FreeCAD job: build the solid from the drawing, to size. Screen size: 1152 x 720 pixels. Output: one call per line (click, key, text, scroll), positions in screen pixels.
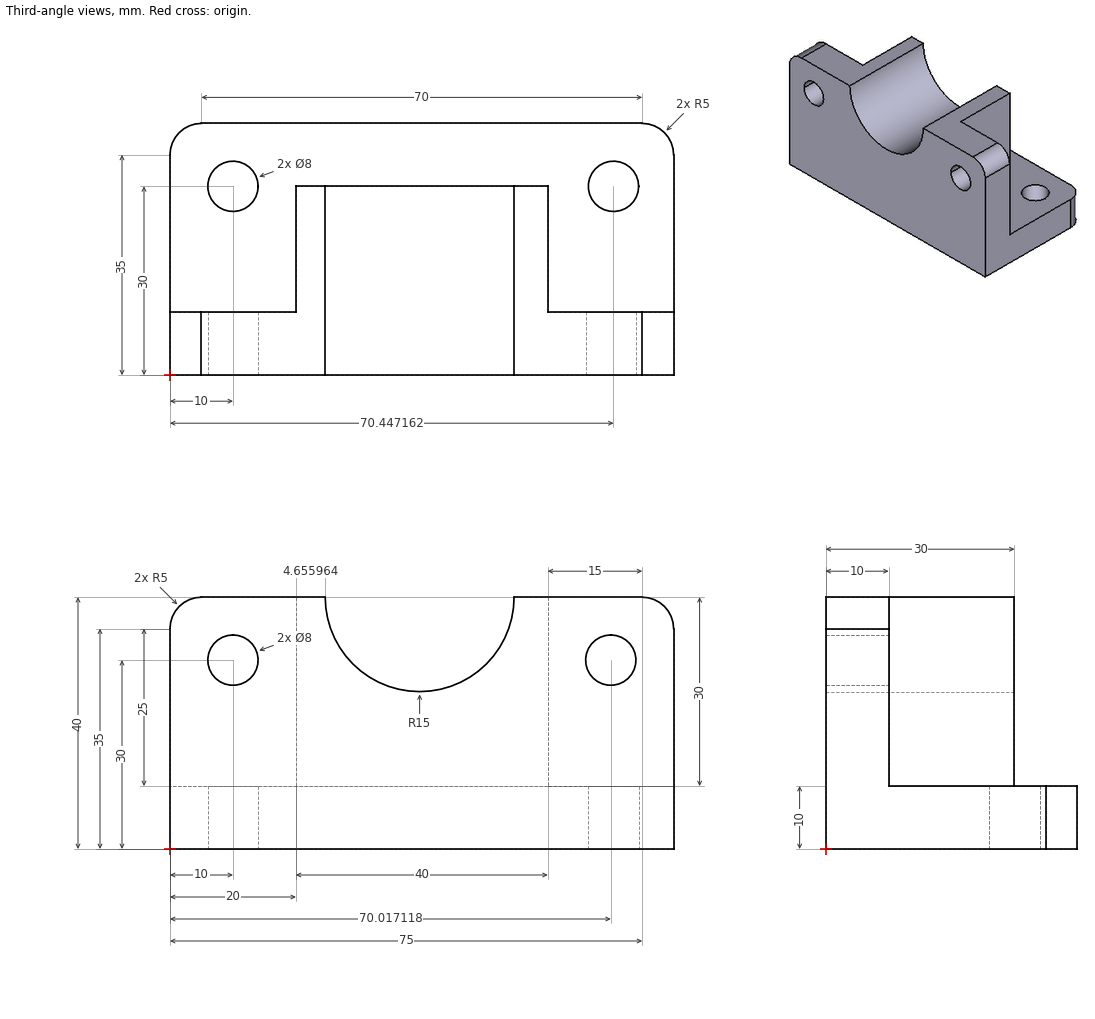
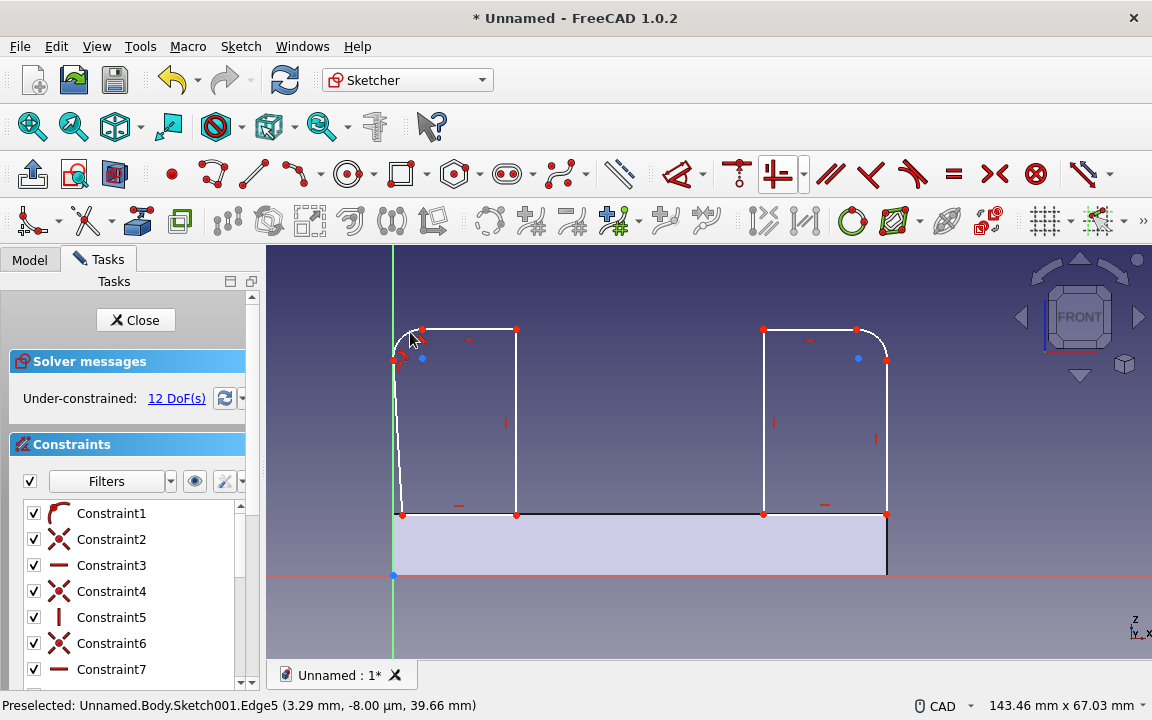
click(829, 330)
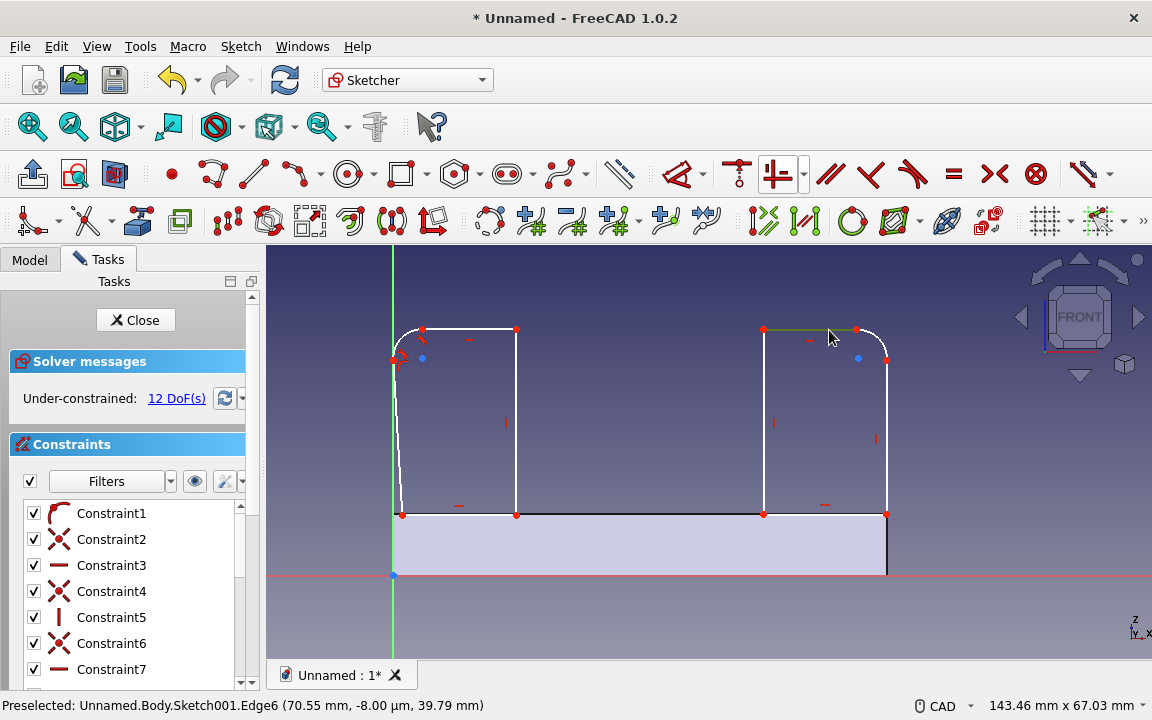
click(884, 347)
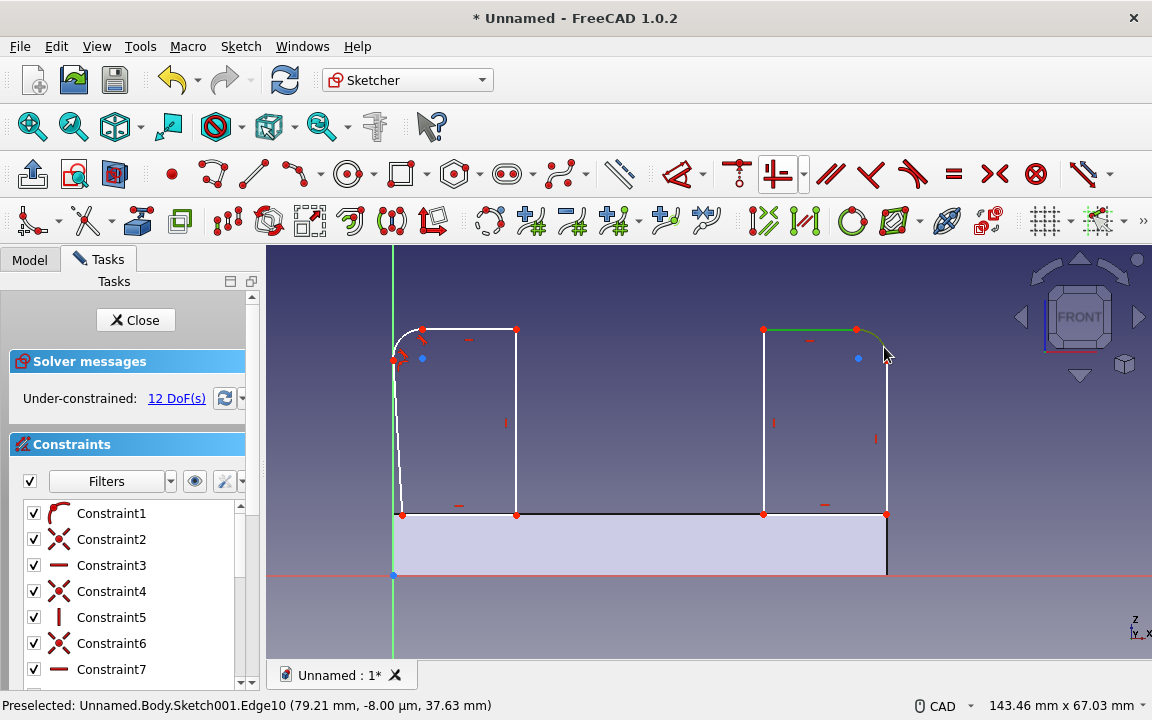
click(913, 174)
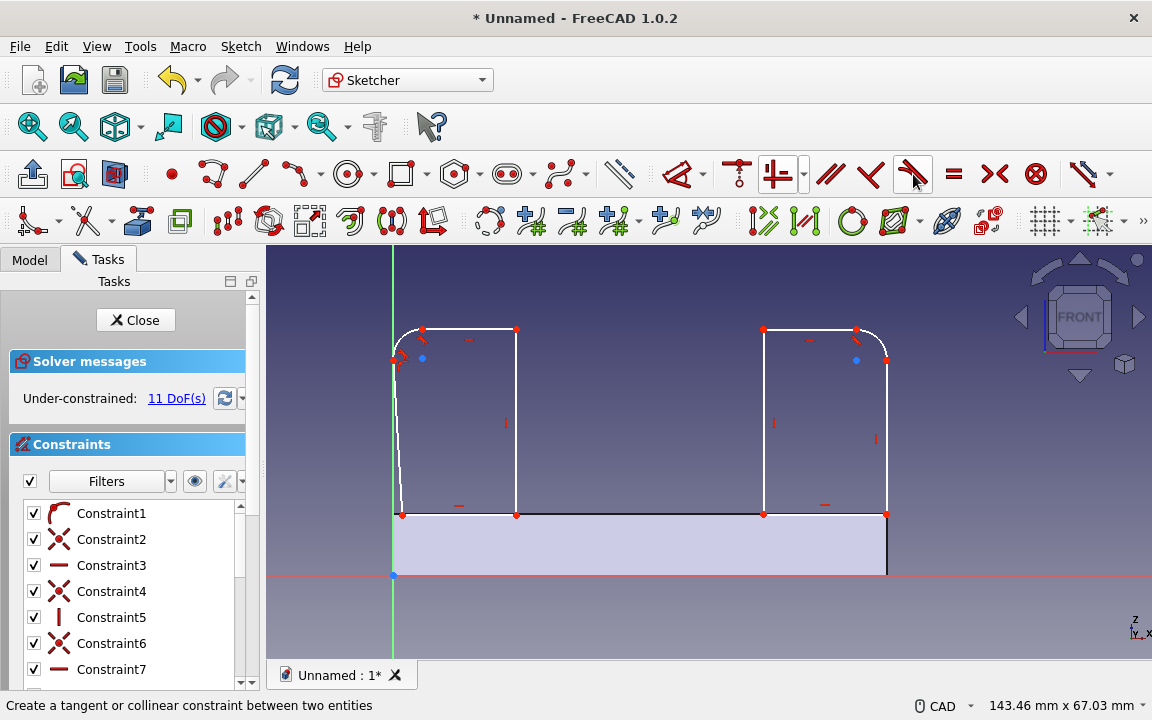
click(887, 469)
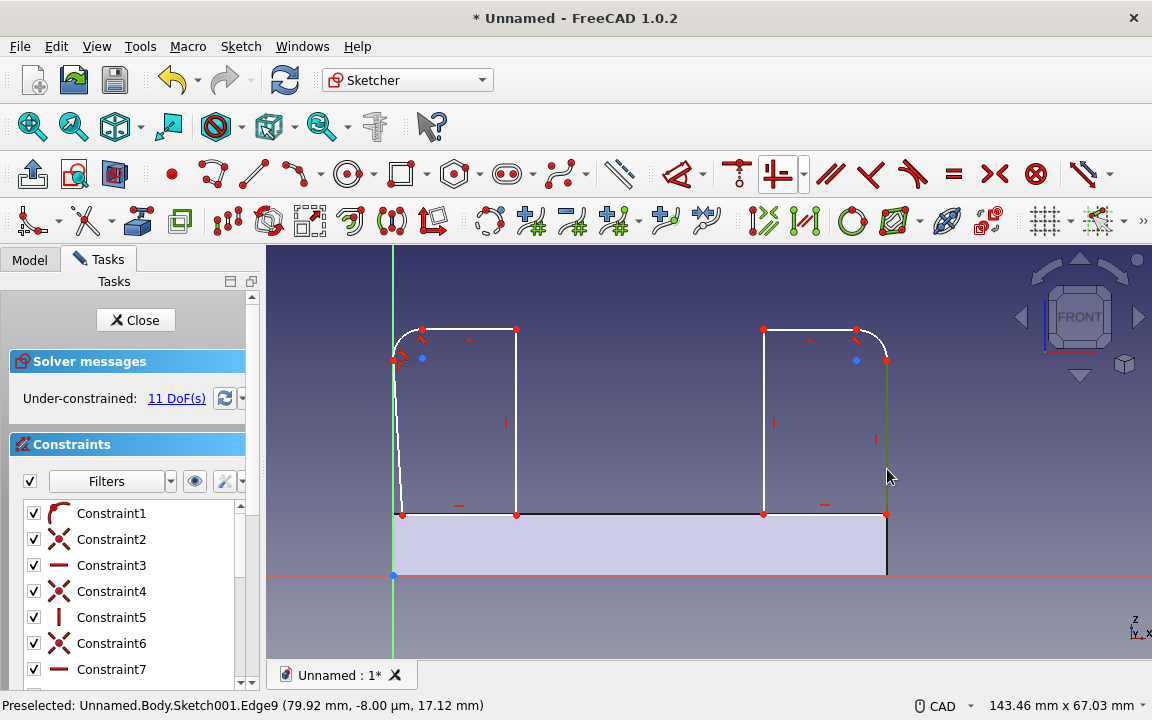
click(884, 347)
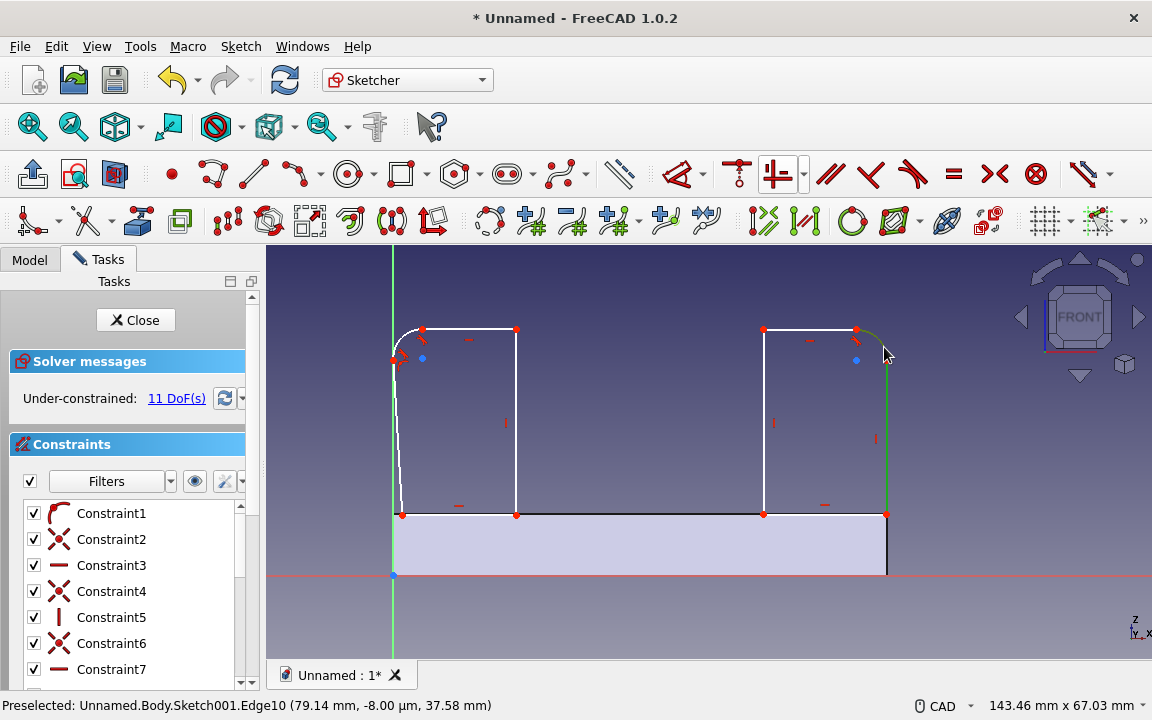
click(913, 174)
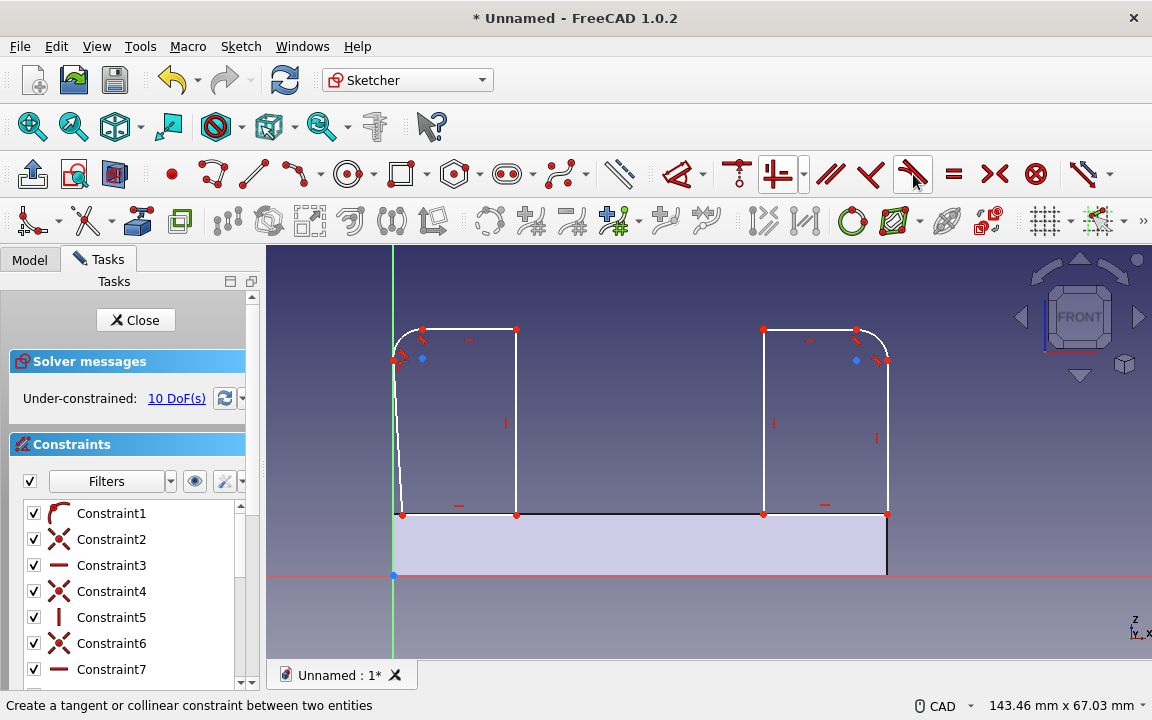
click(396, 407)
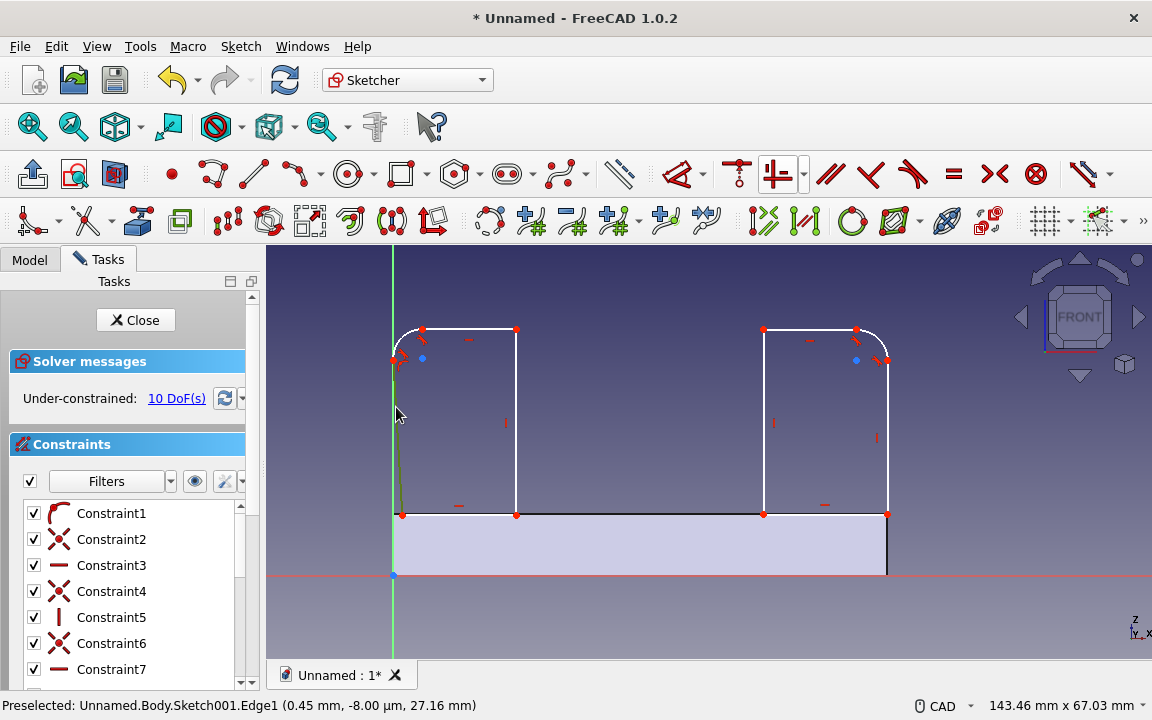
key(v)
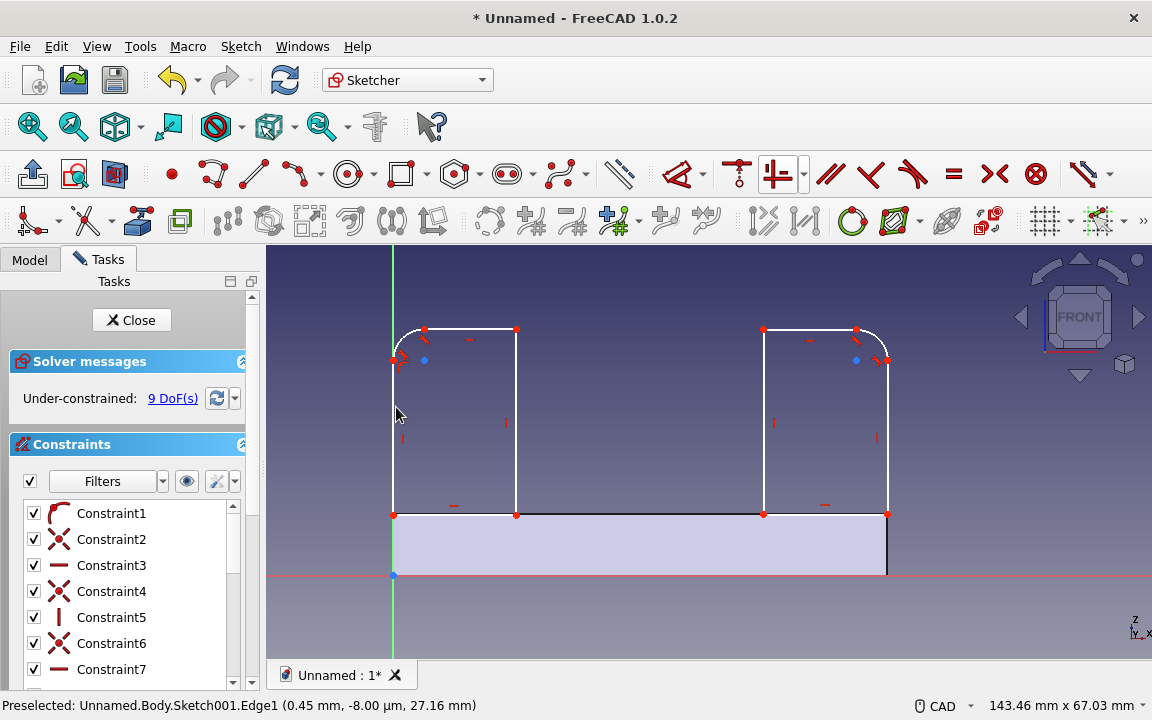
click(410, 333)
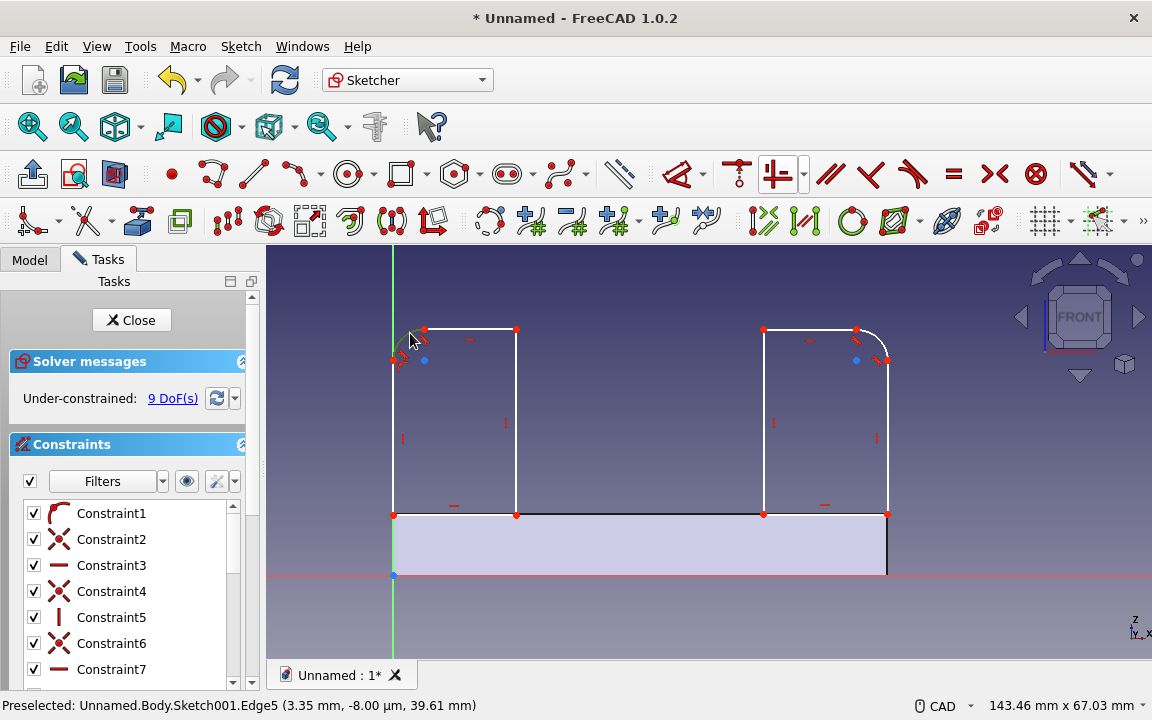
click(885, 347)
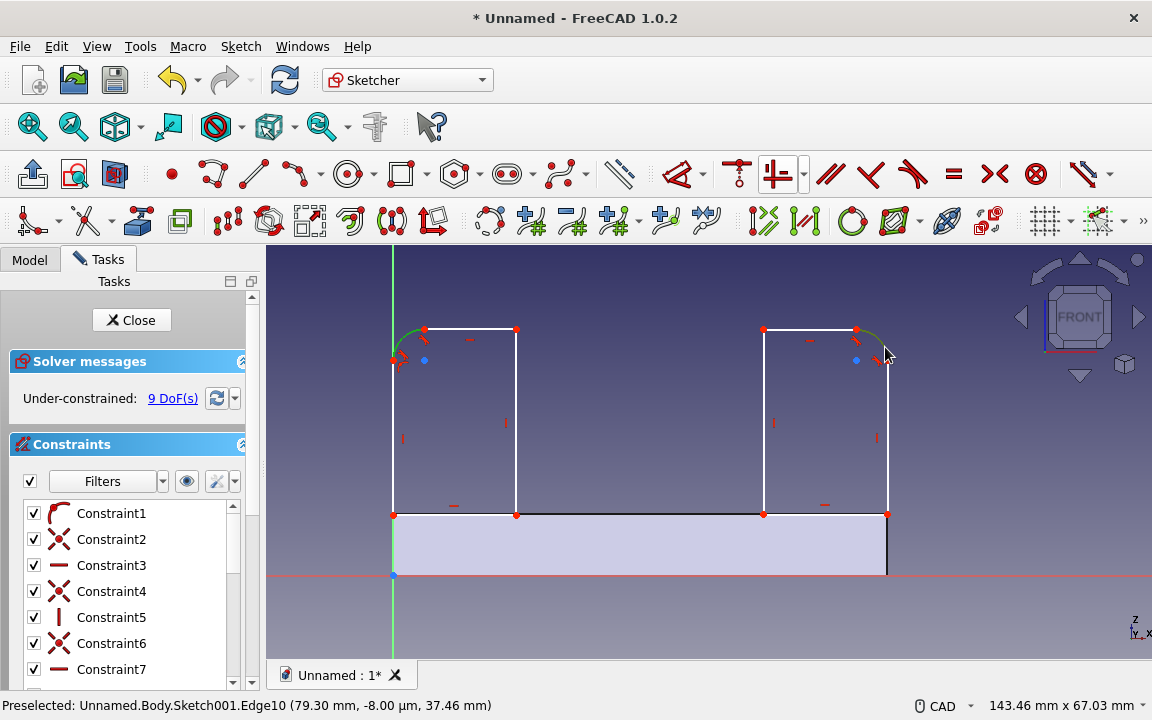
click(954, 174)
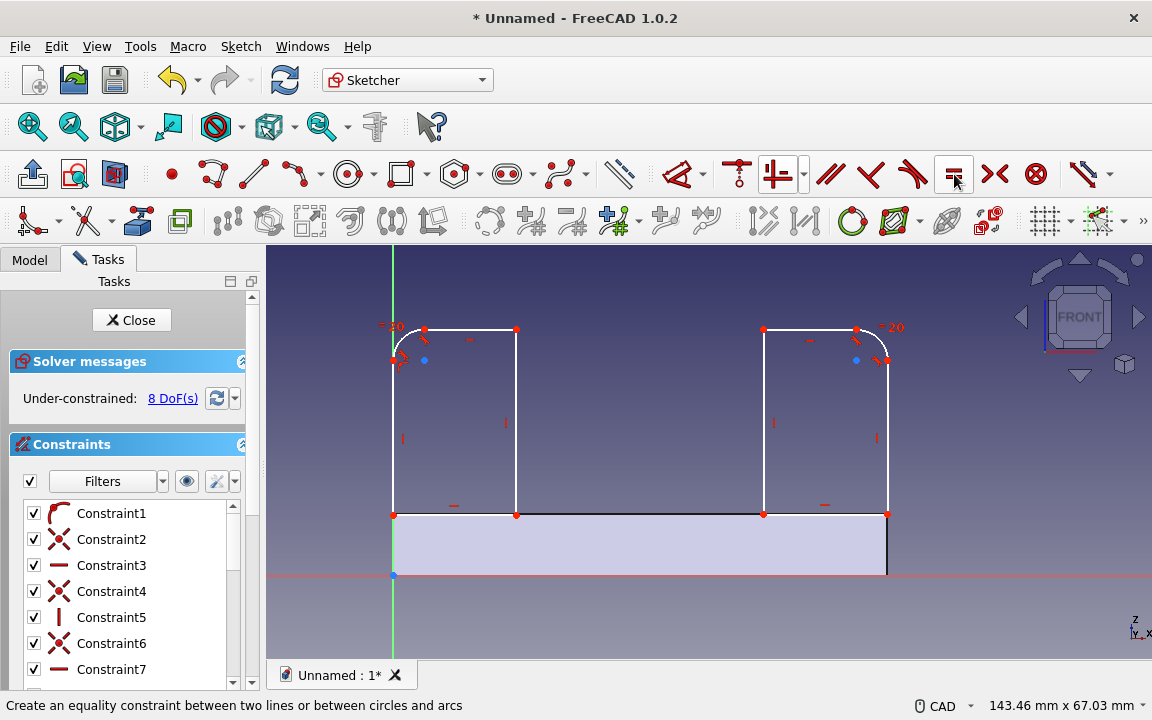
click(676, 174)